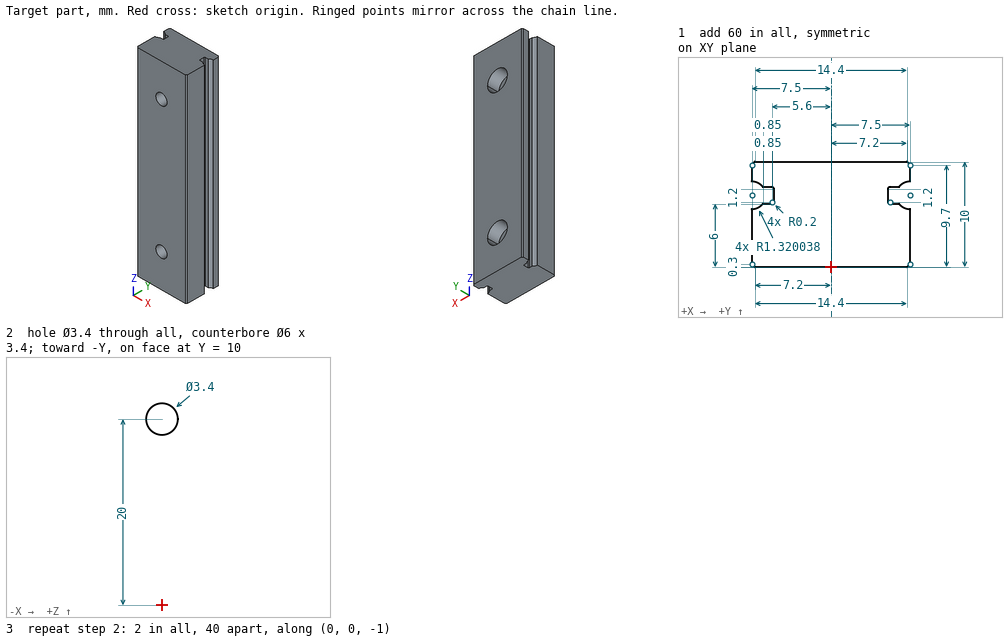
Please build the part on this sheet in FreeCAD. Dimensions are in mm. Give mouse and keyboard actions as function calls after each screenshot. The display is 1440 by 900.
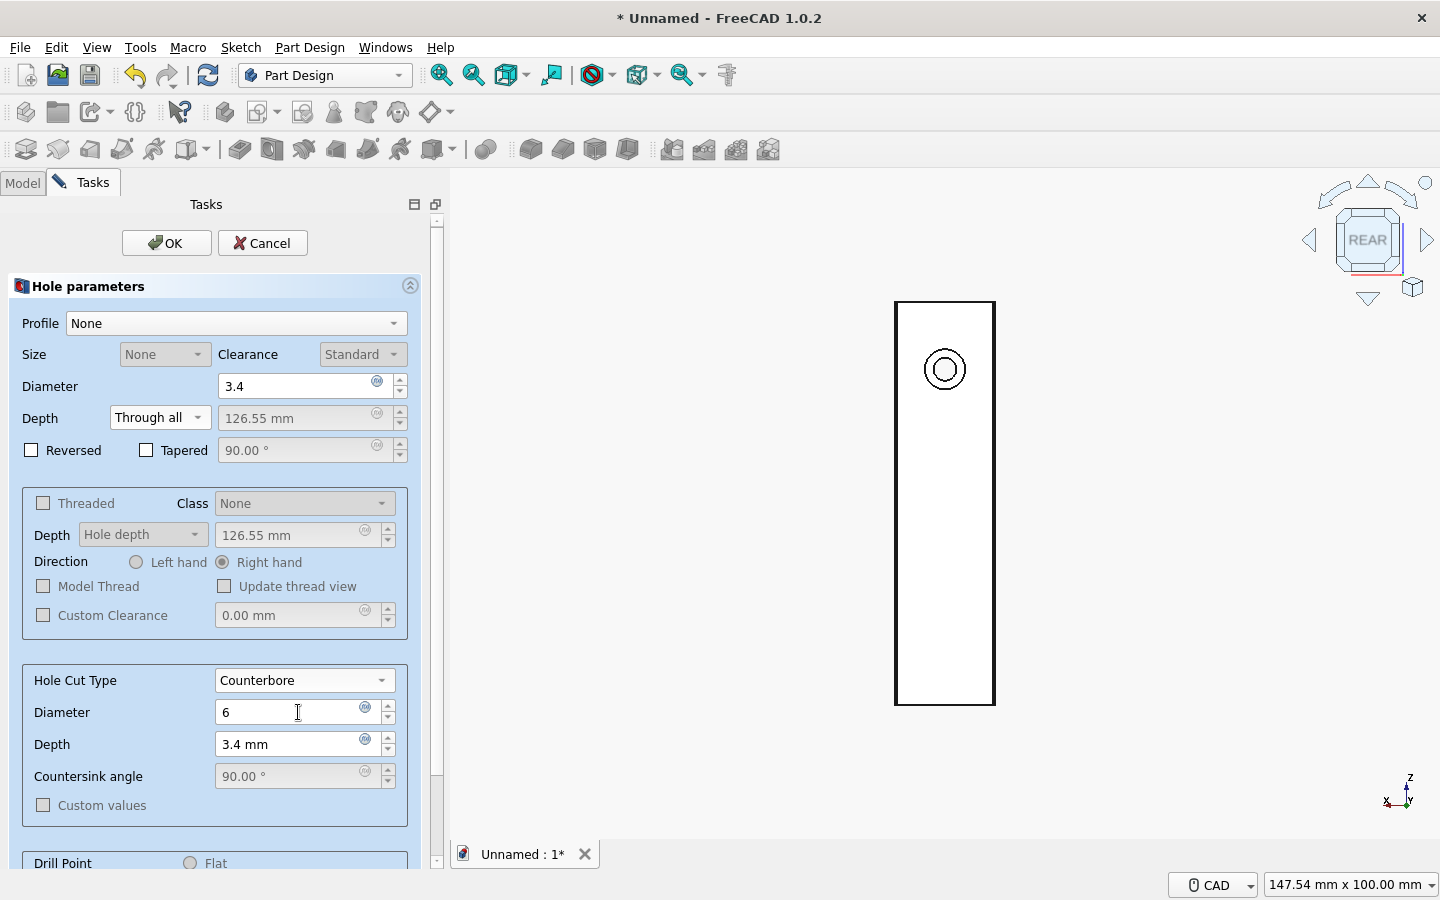
click(167, 243)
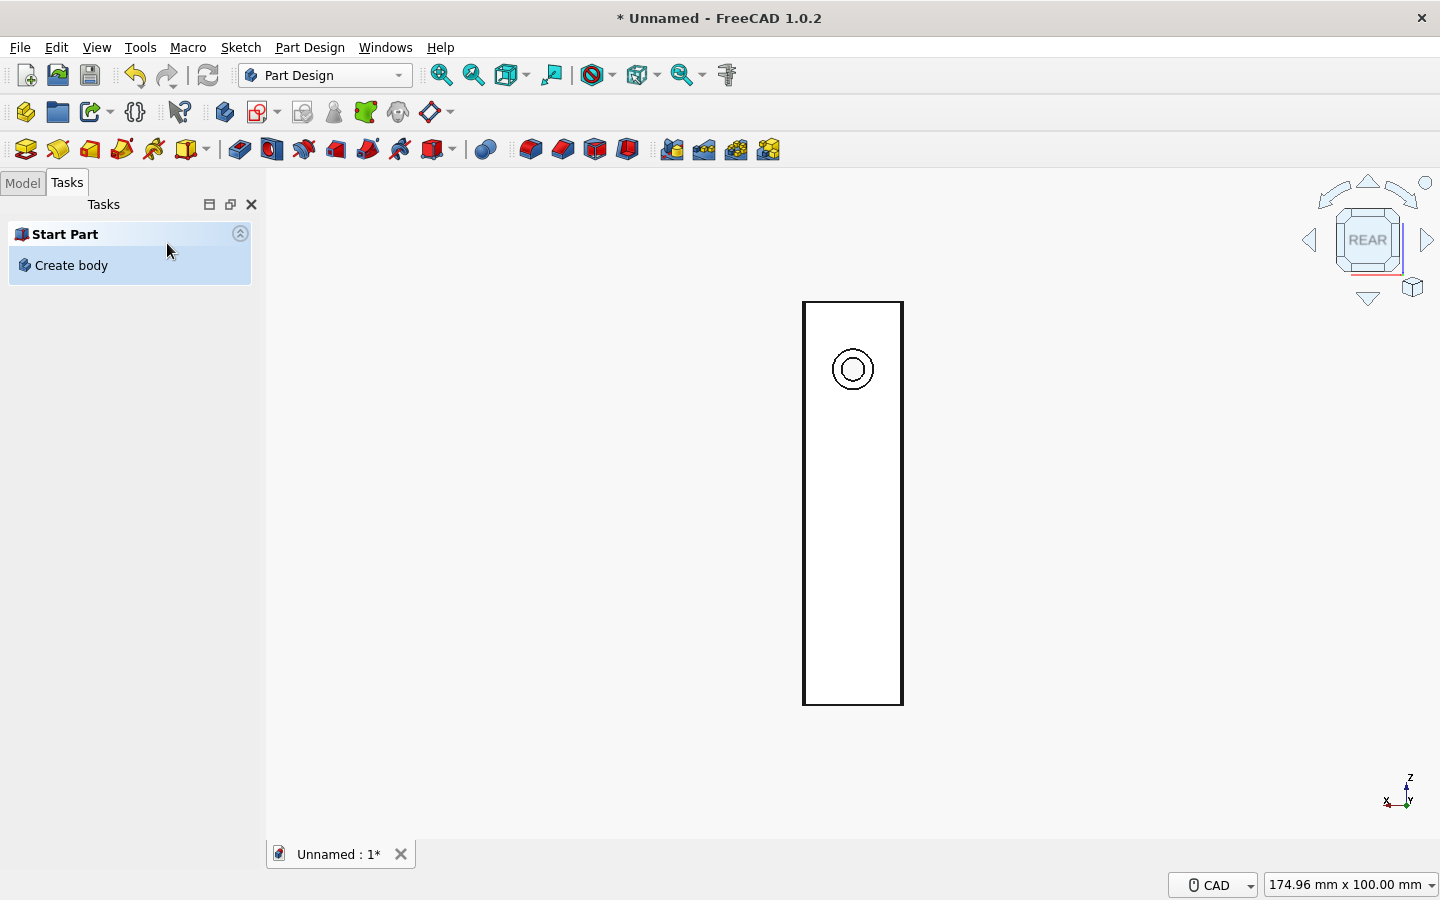
click(23, 182)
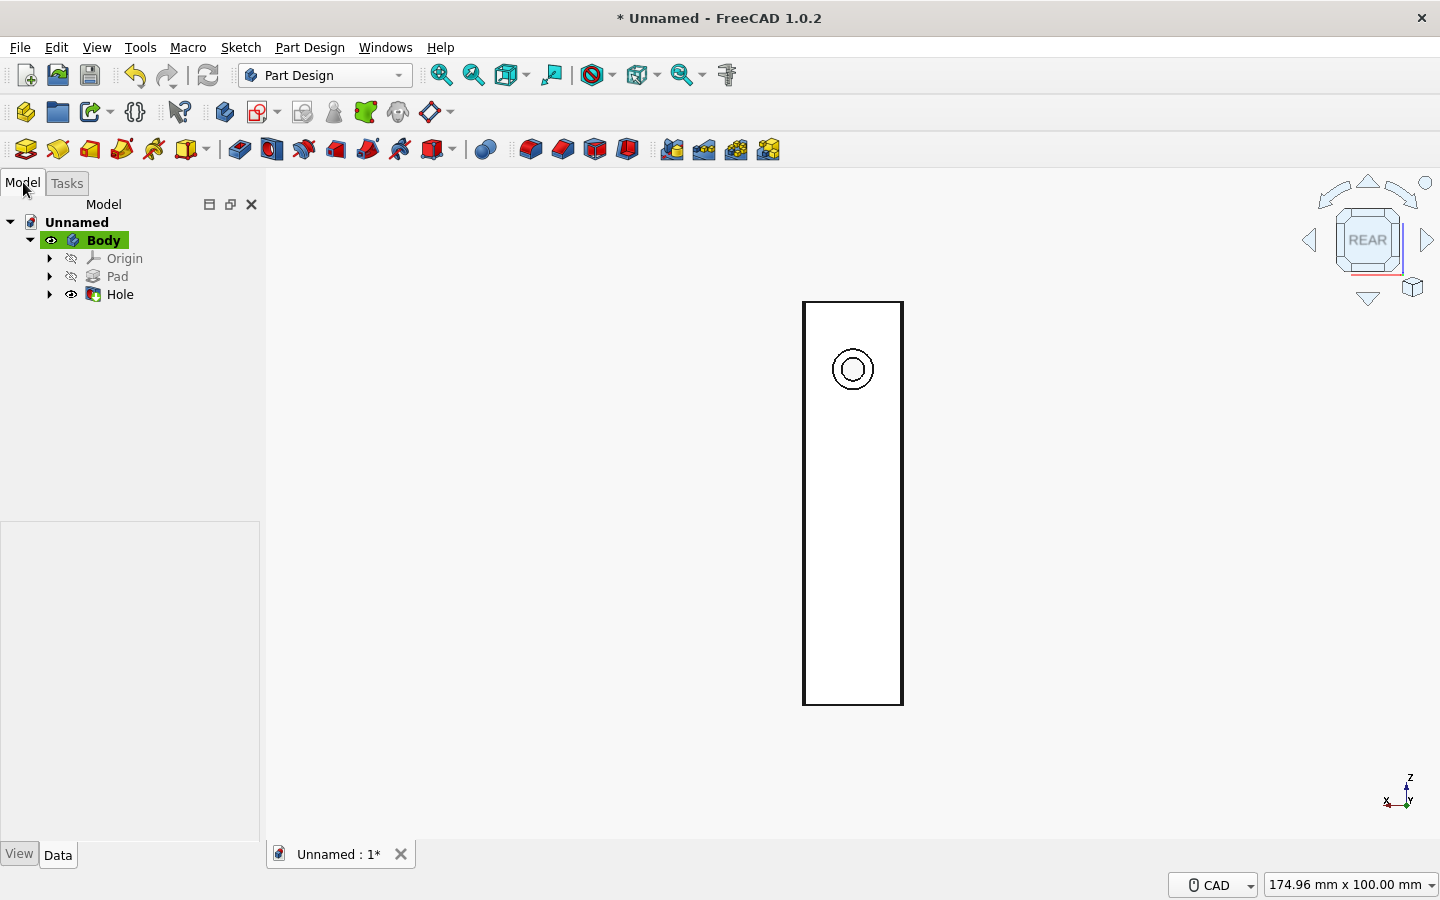
click(116, 294)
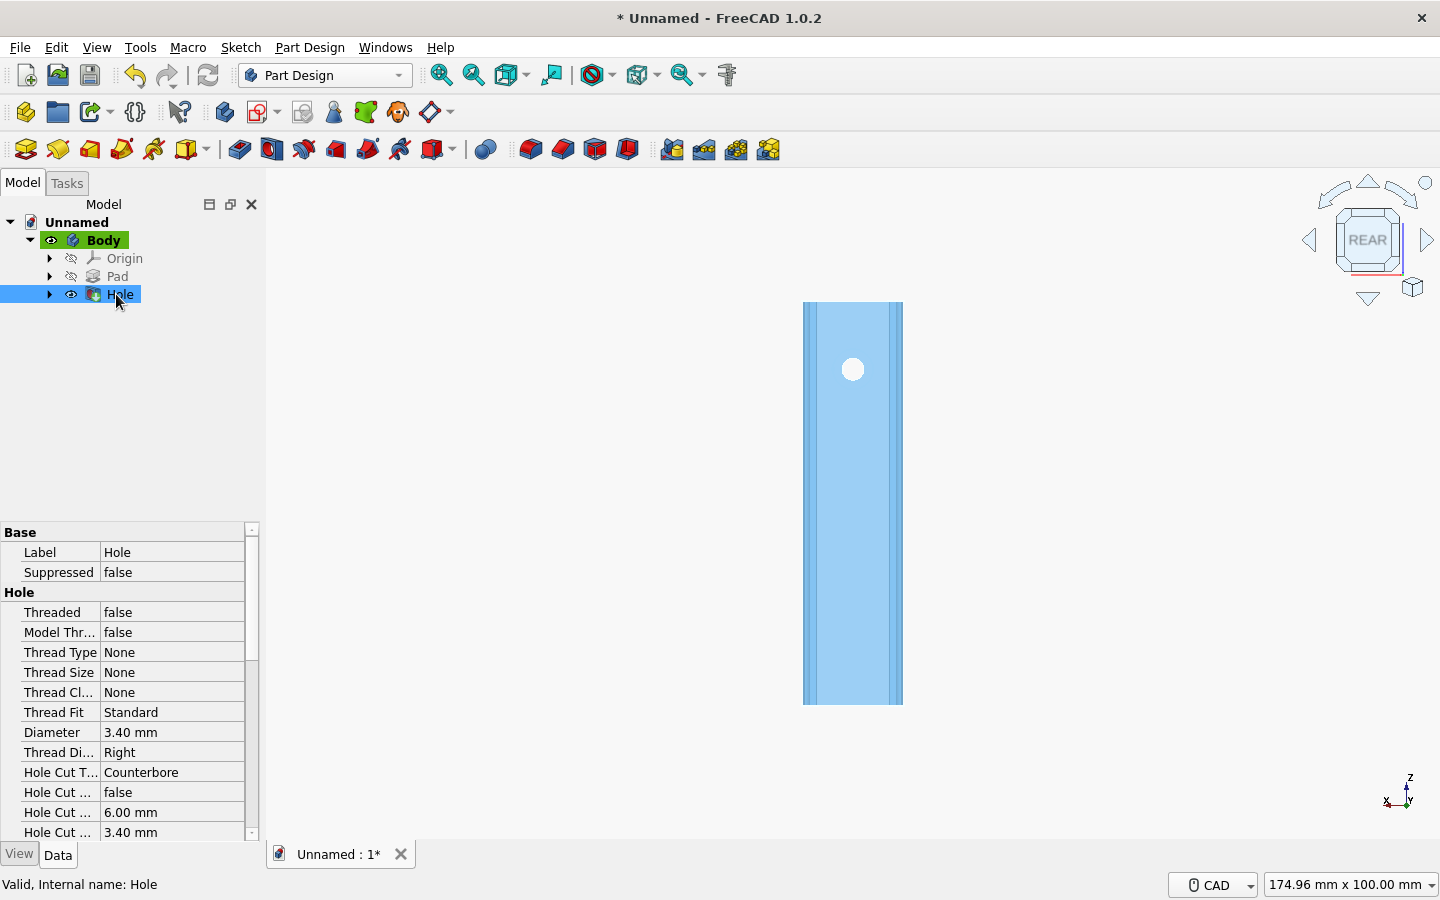
click(704, 150)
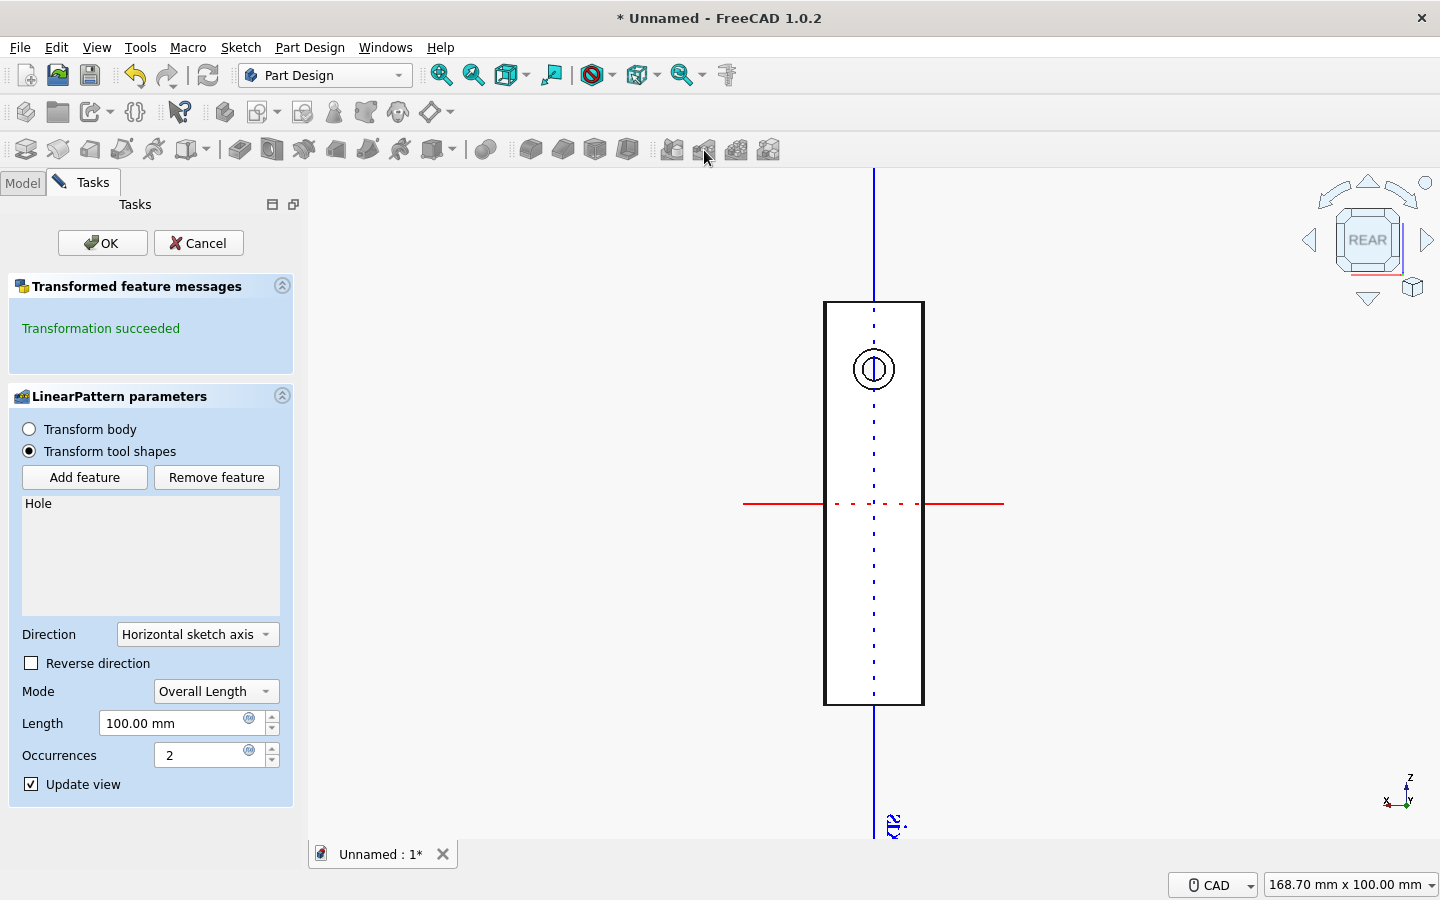
click(198, 634)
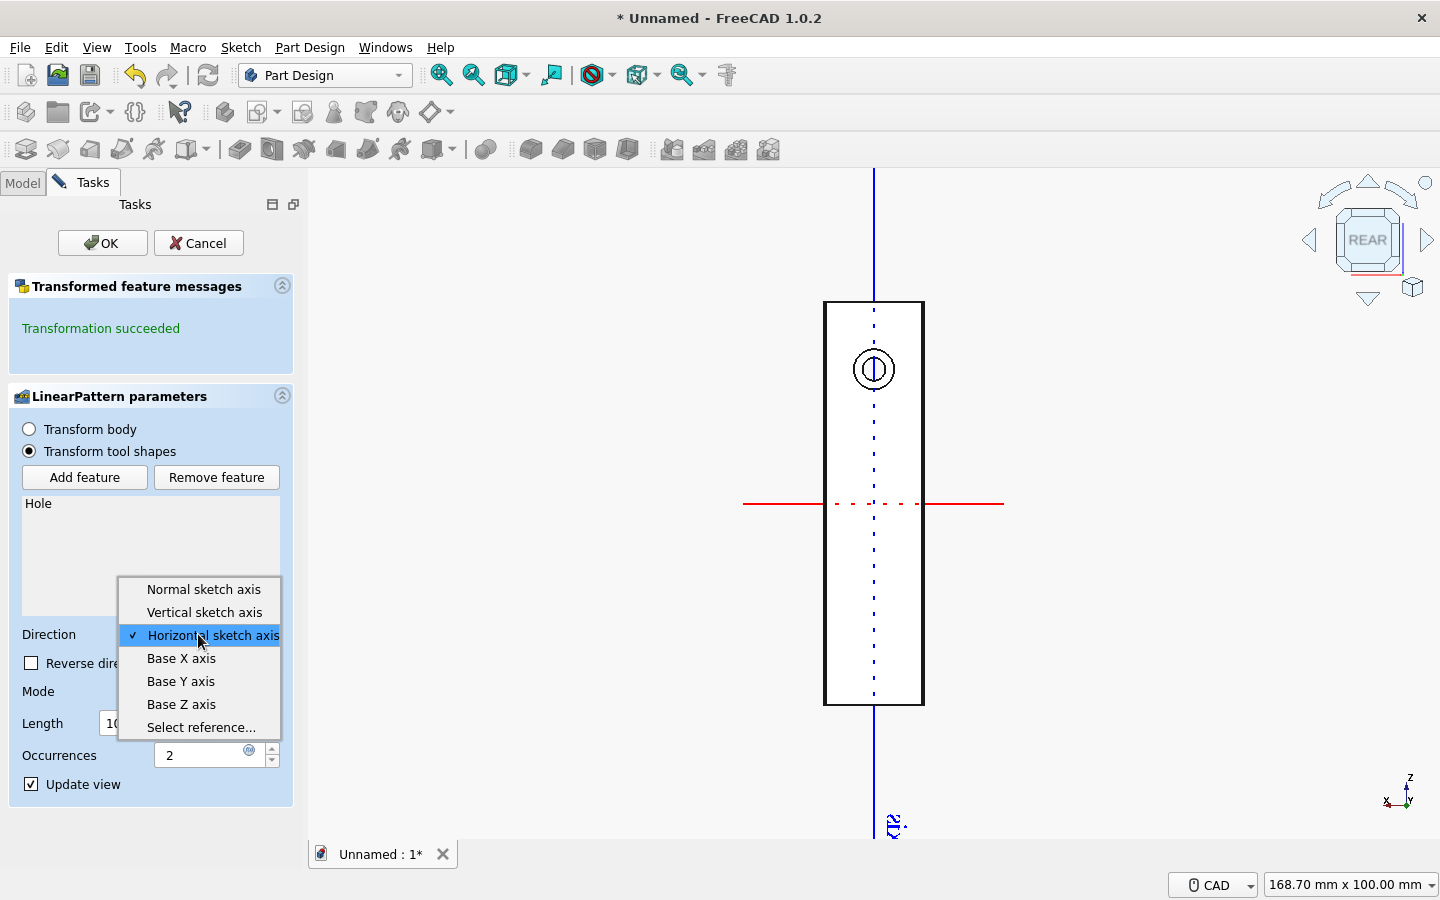
click(198, 704)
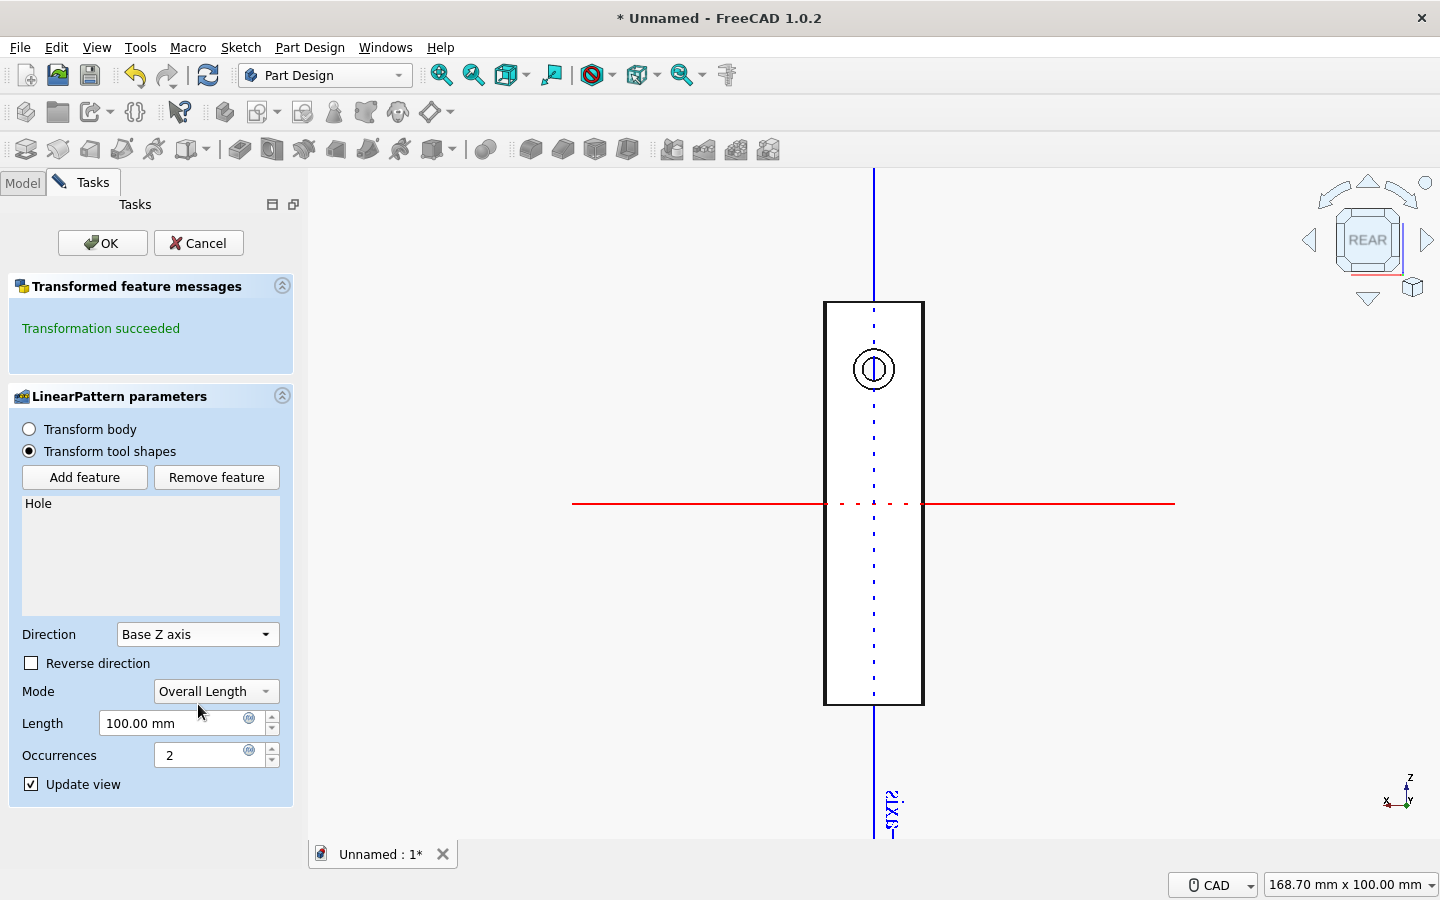
click(217, 692)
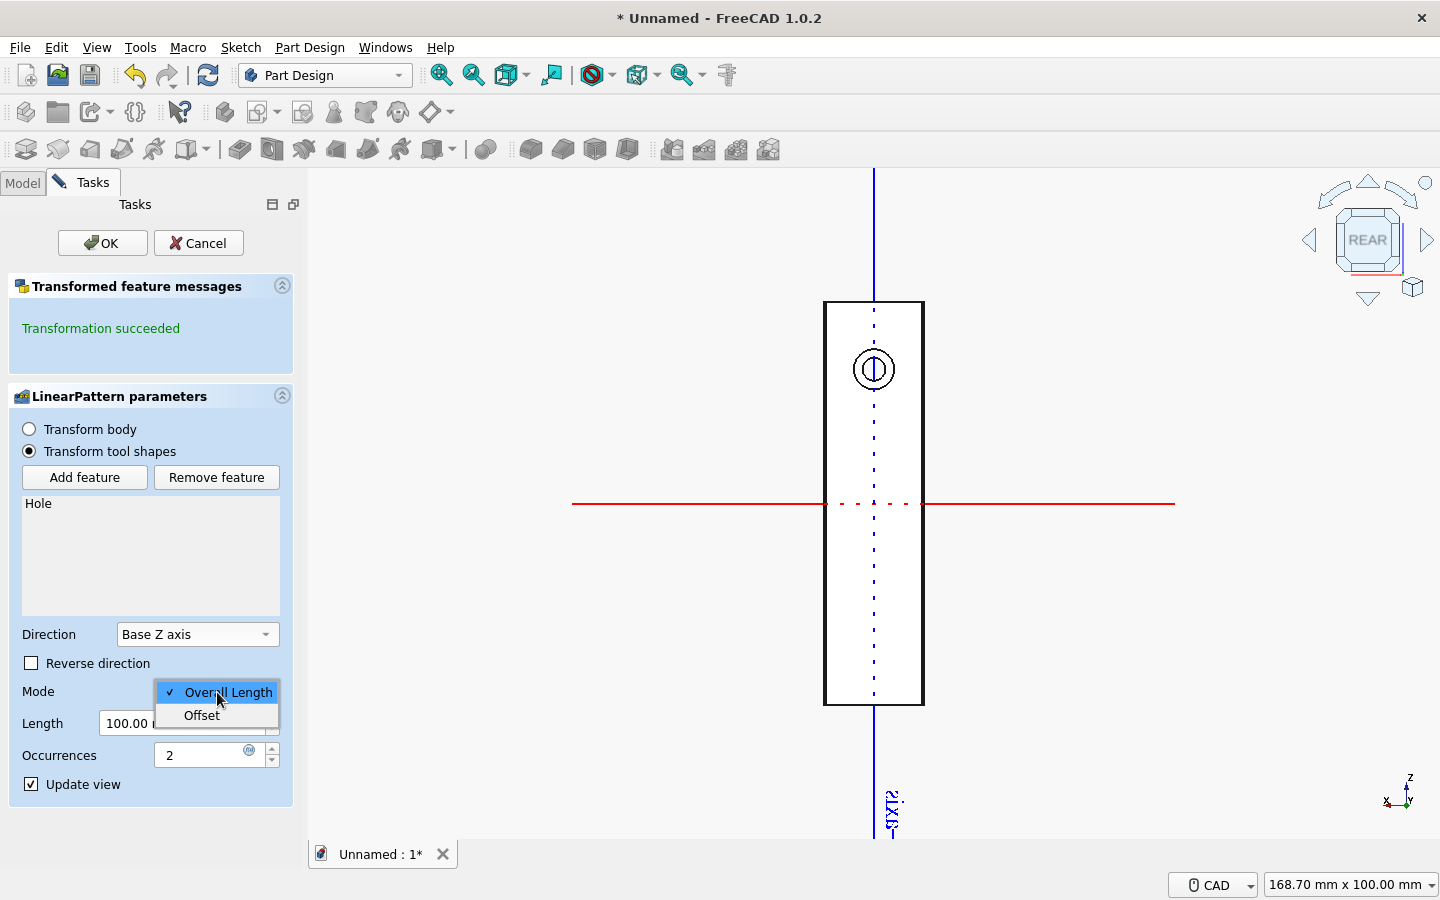
click(216, 716)